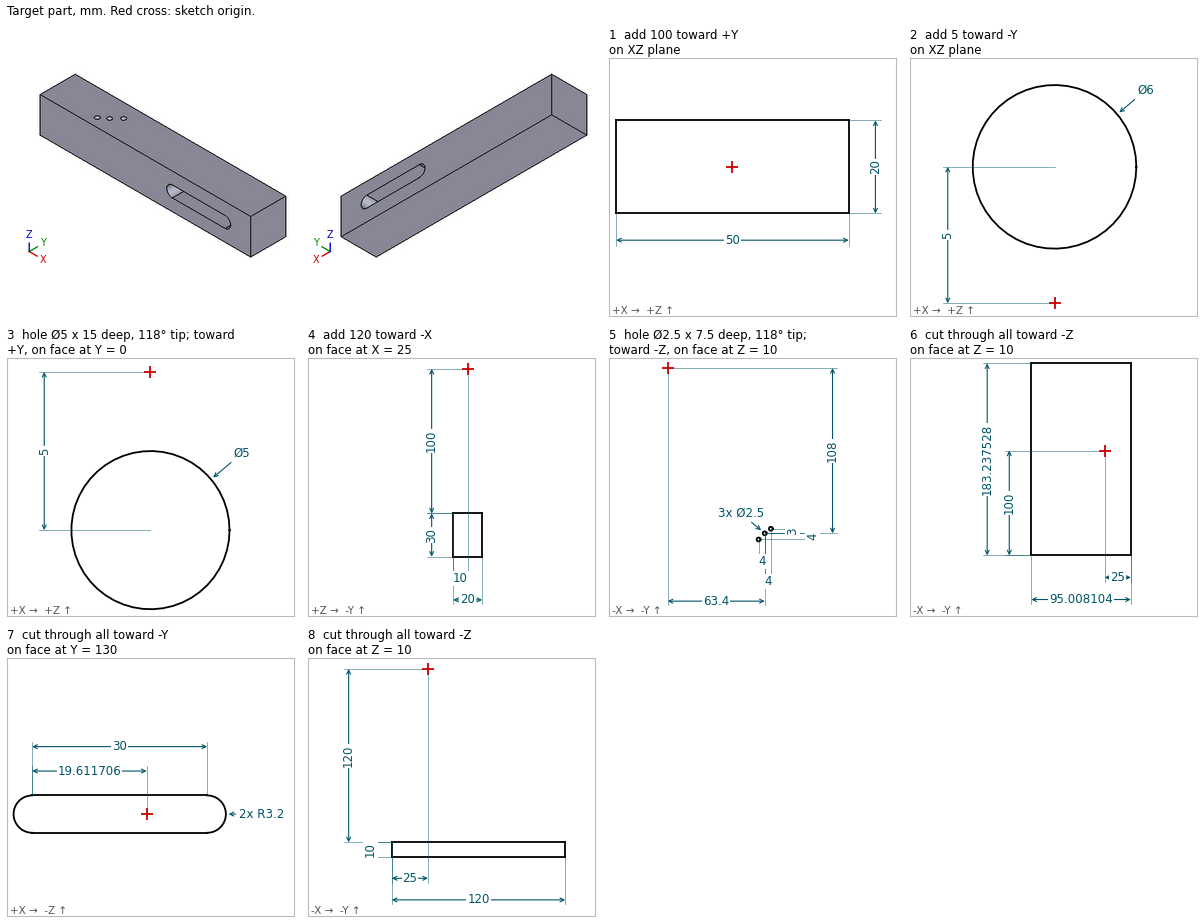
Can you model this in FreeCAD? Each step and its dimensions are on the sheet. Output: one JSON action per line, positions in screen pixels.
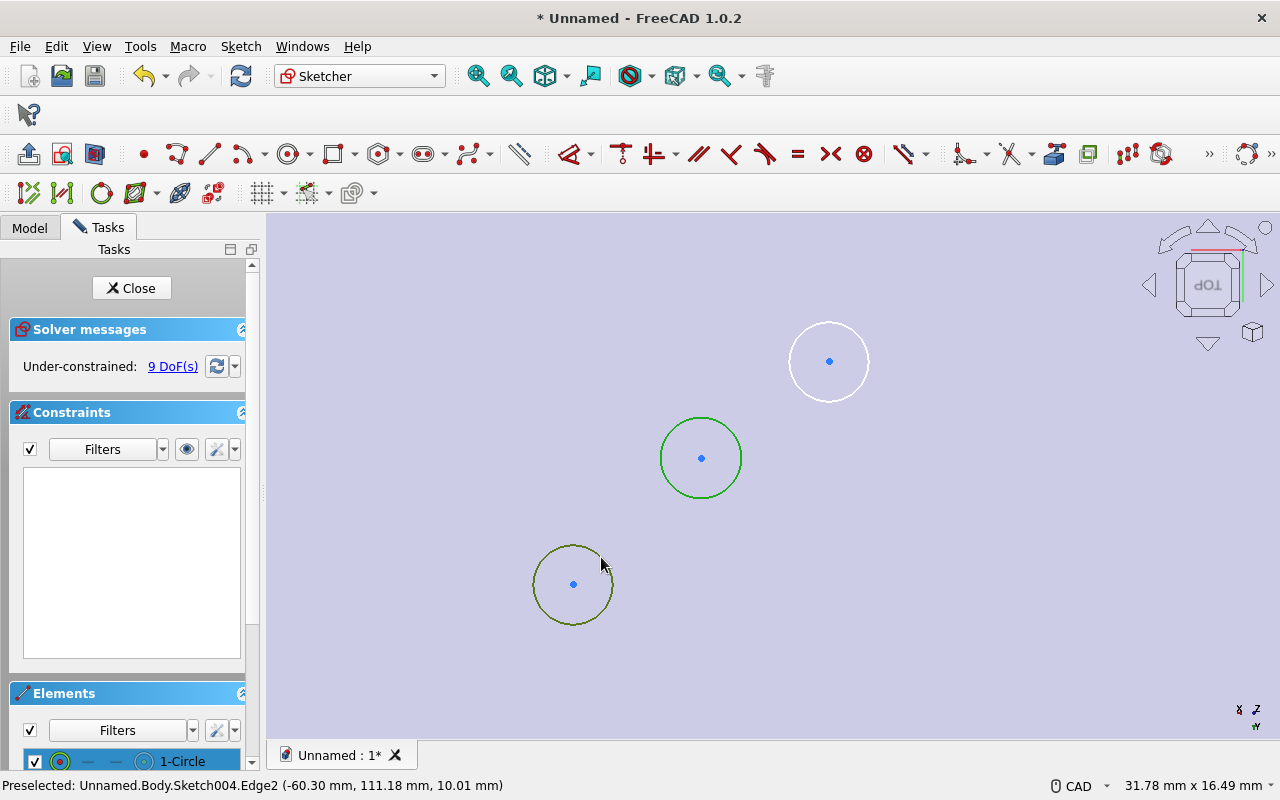
{"action": "left_click", "coordinate": [857, 334]}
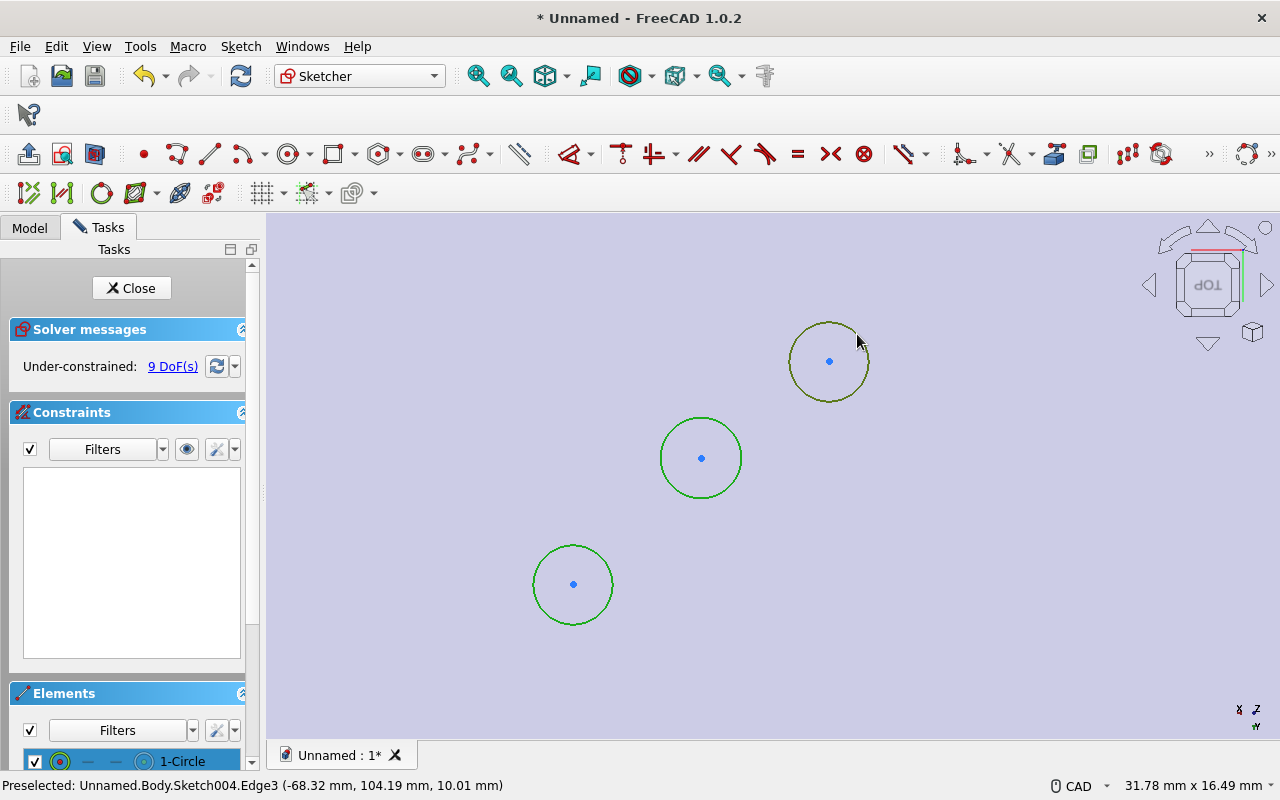
{"action": "key", "text": "e"}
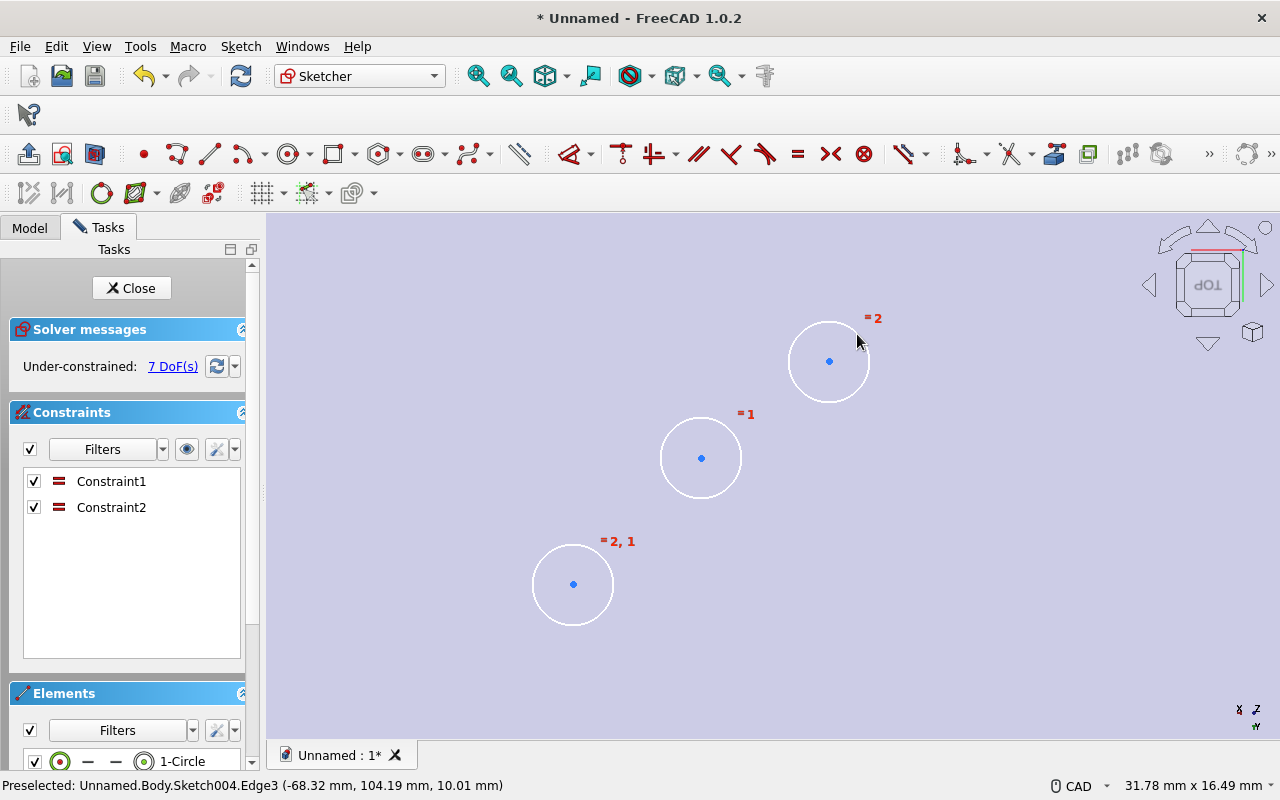
{"action": "left_click", "coordinate": [568, 154]}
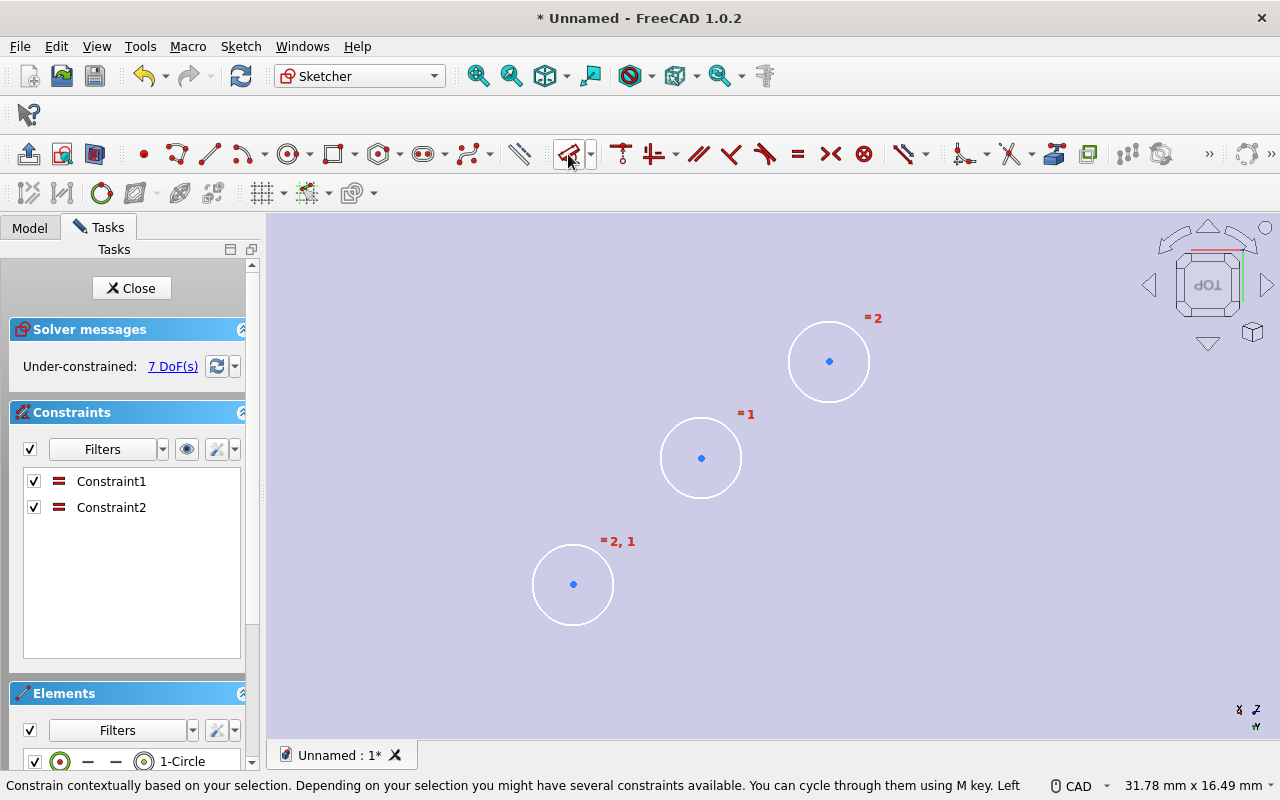
{"action": "left_click", "coordinate": [729, 429]}
{"action": "left_click", "coordinate": [751, 406]}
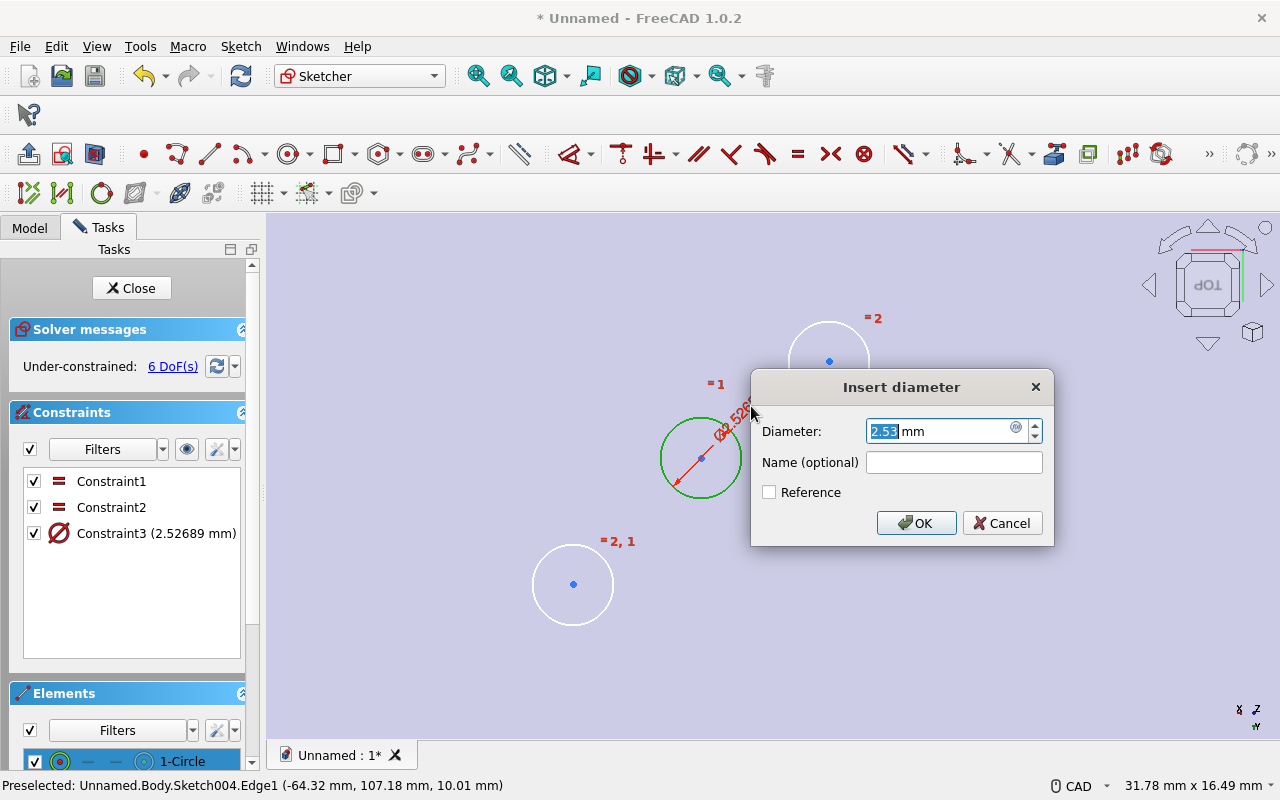
{"action": "type", "text": "2.5"}
{"action": "key", "text": "Return"}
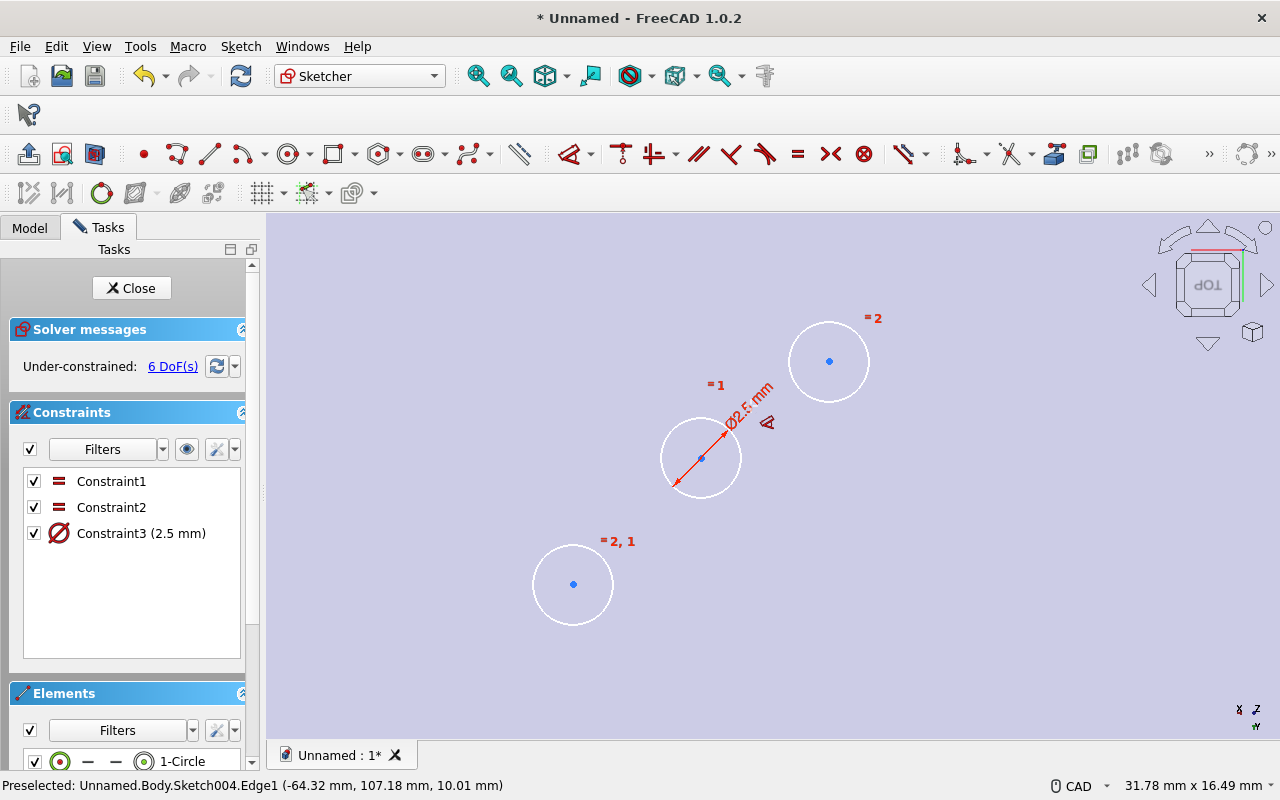
{"action": "left_click", "coordinate": [701, 458]}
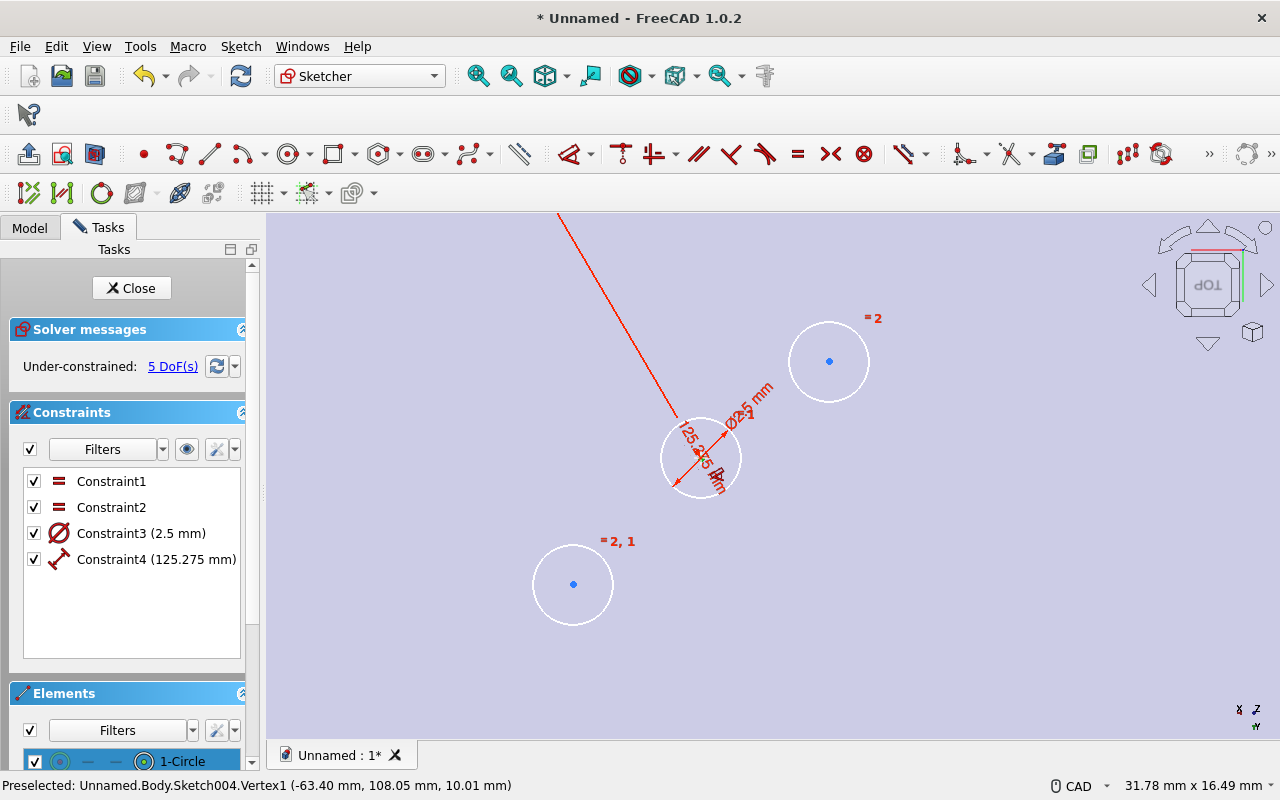
{"action": "left_click", "coordinate": [573, 585]}
{"action": "left_click", "coordinate": [637, 619]}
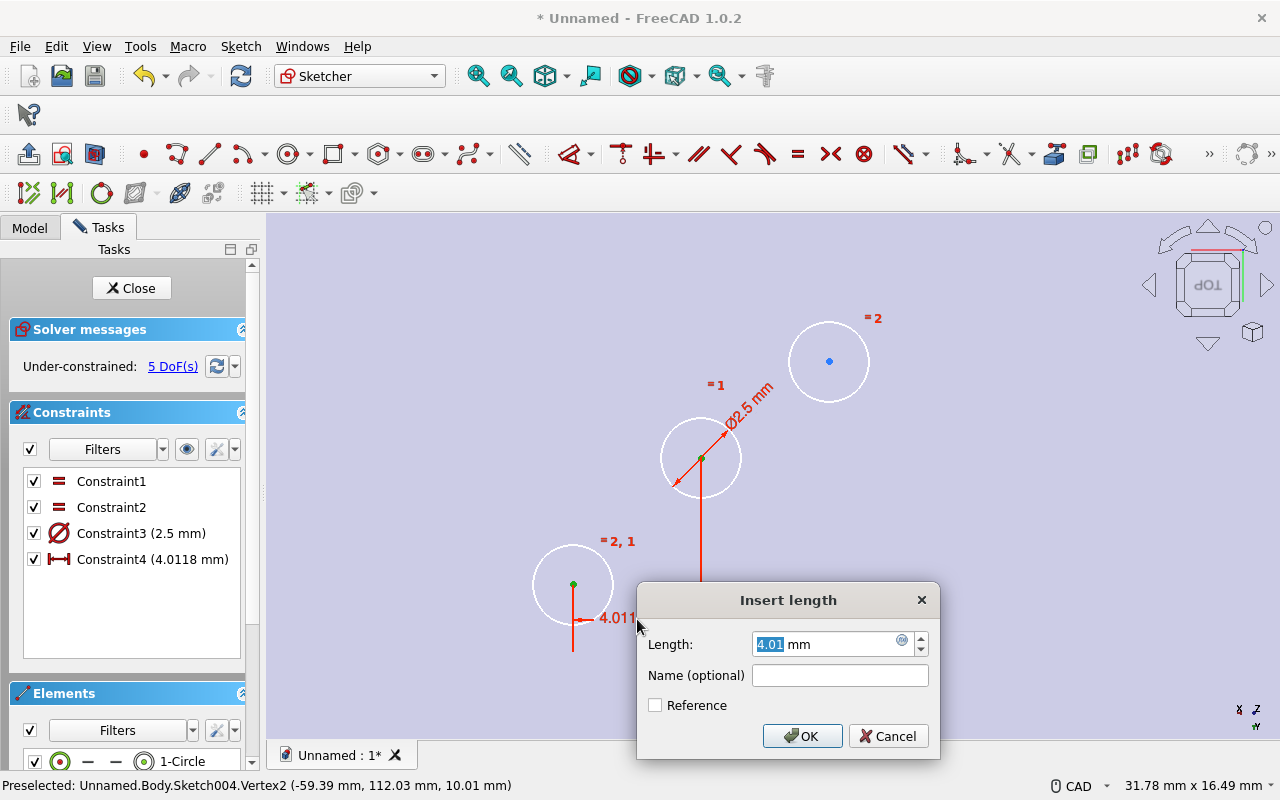
{"action": "type", "text": "4"}
{"action": "key", "text": "Return"}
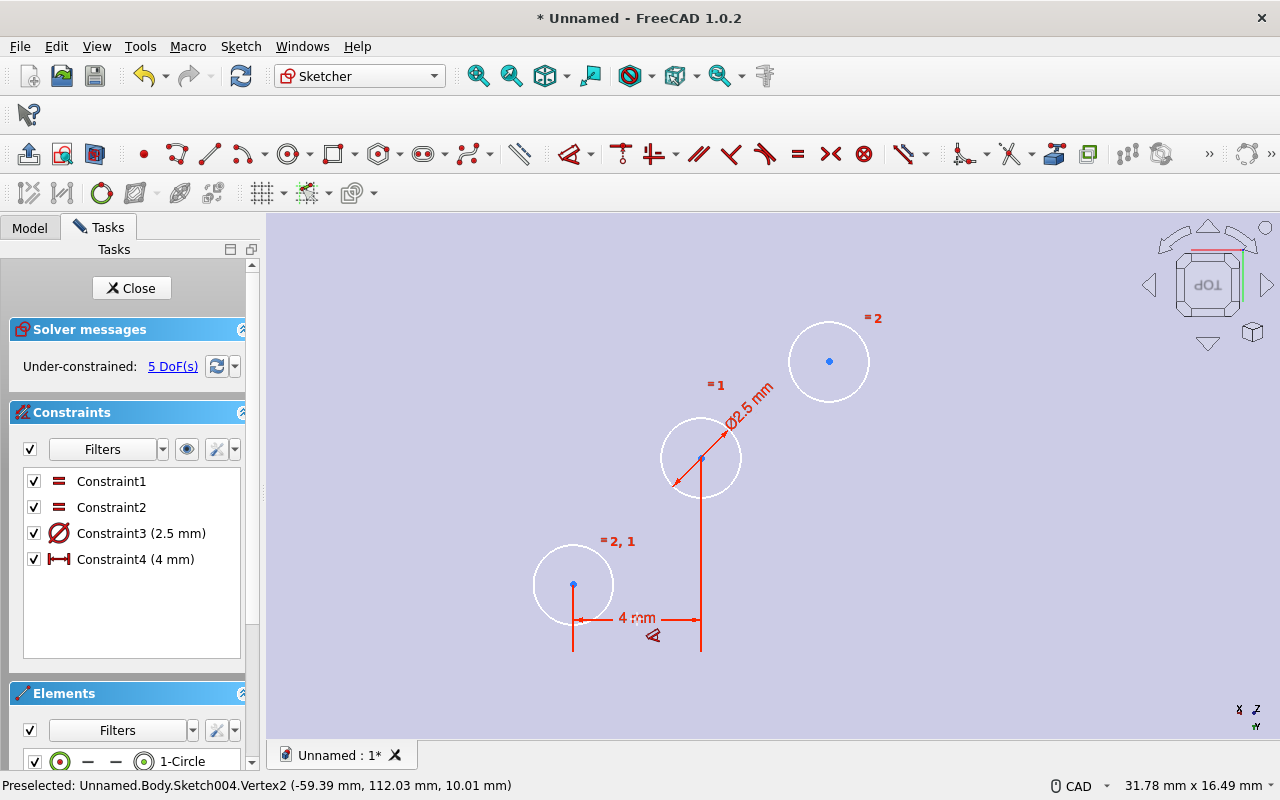
{"action": "left_click", "coordinate": [701, 458]}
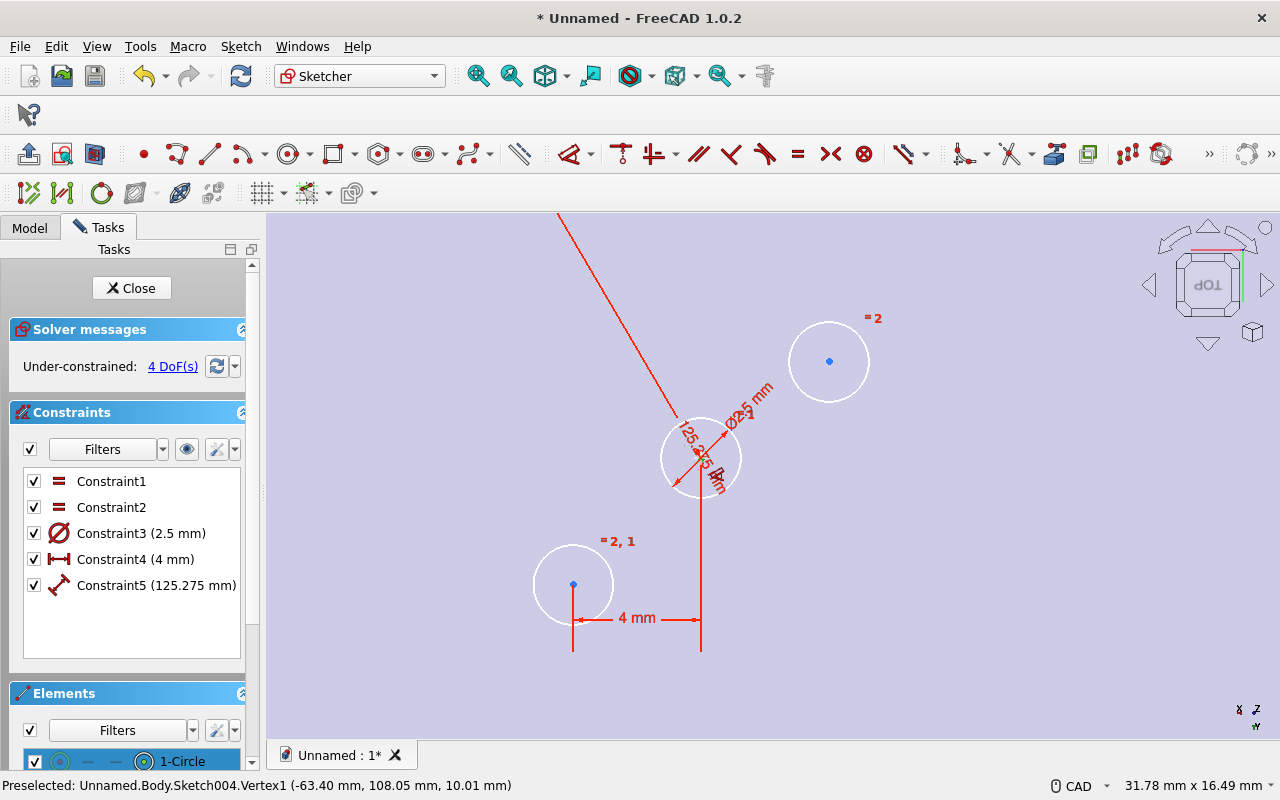
{"action": "left_click", "coordinate": [573, 585]}
{"action": "left_click", "coordinate": [539, 522]}